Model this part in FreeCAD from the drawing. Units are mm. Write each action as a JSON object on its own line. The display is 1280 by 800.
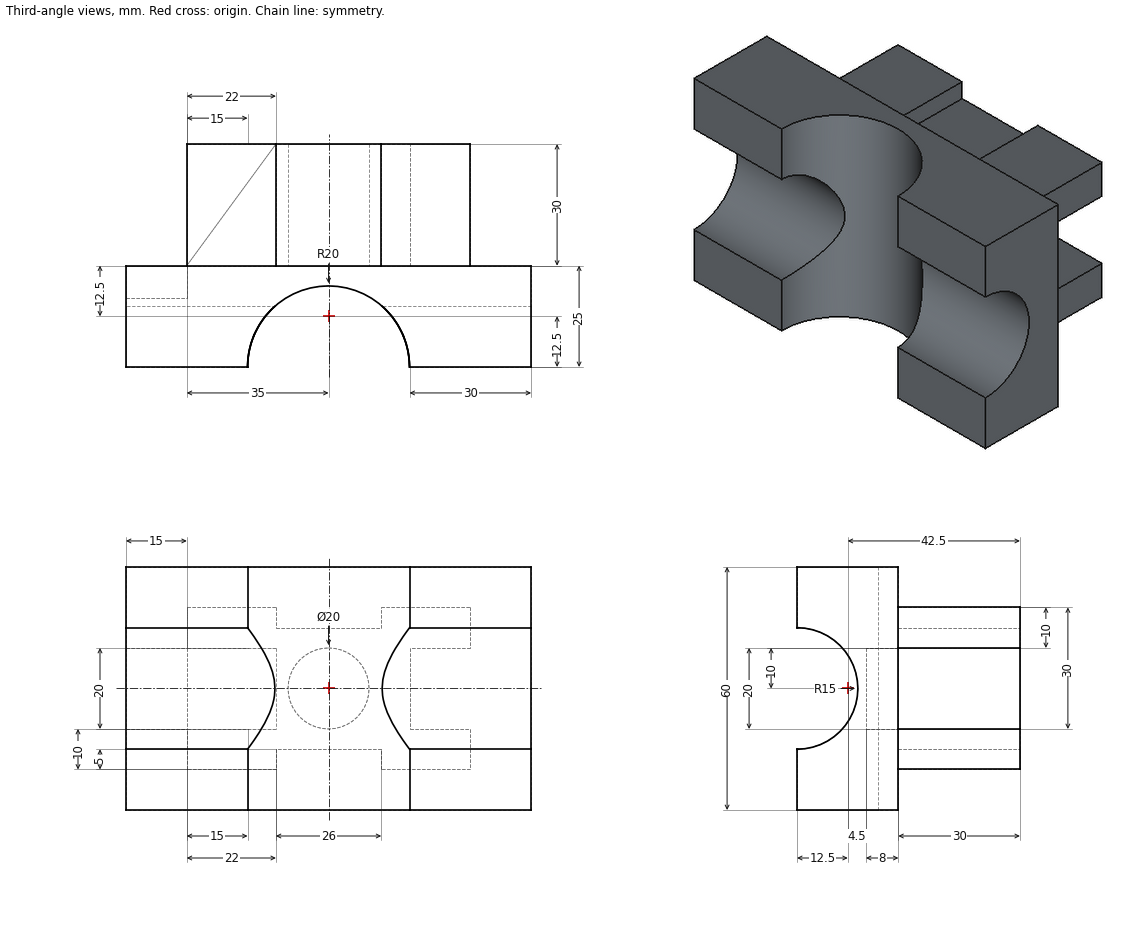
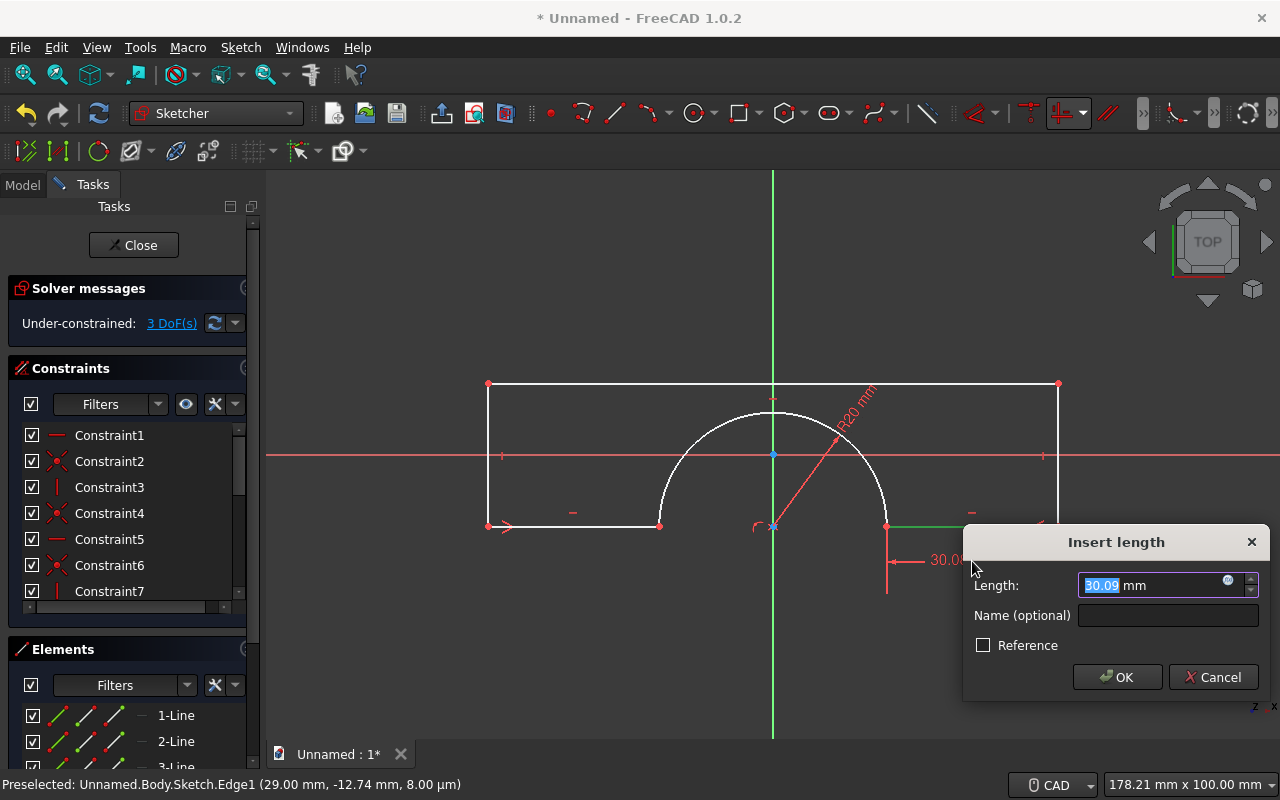
{"action": "type", "text": "30"}
{"action": "key", "text": "Return"}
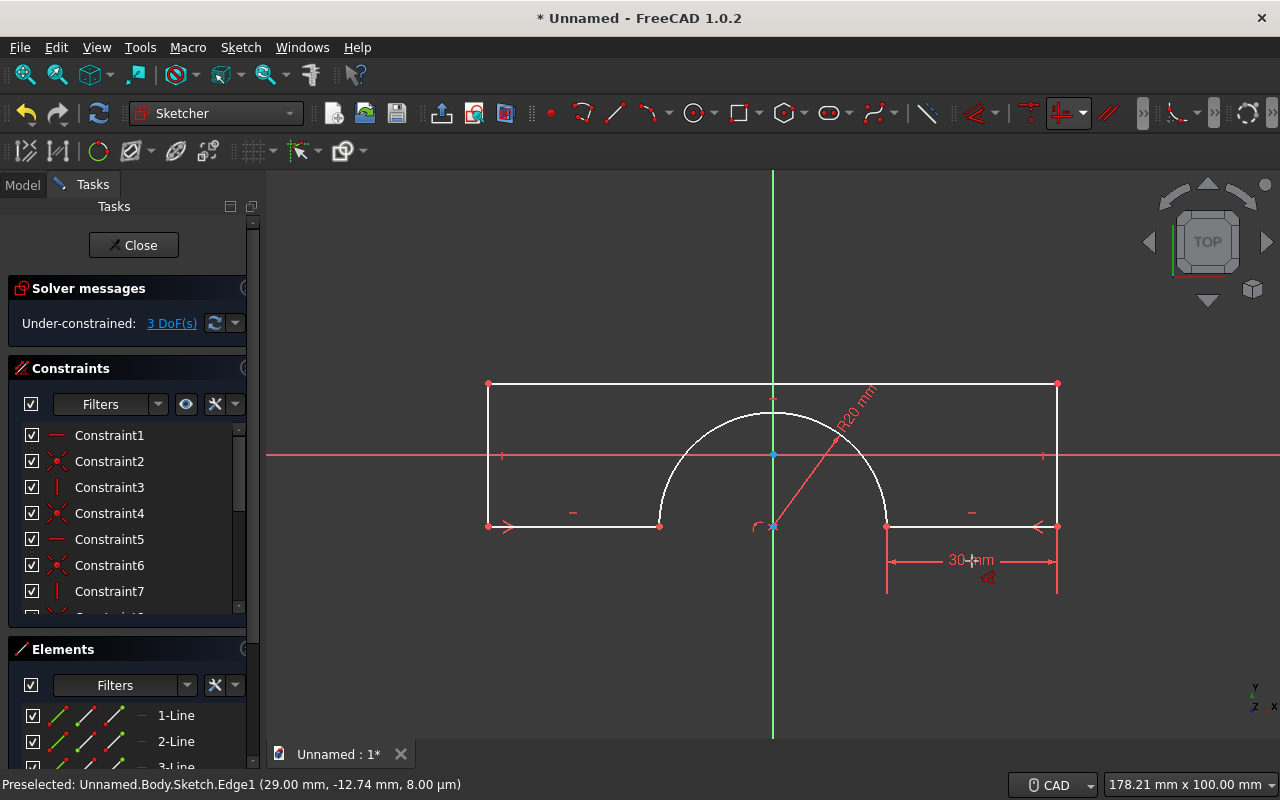
{"action": "left_click", "coordinate": [1057, 484]}
{"action": "left_click", "coordinate": [1091, 423]}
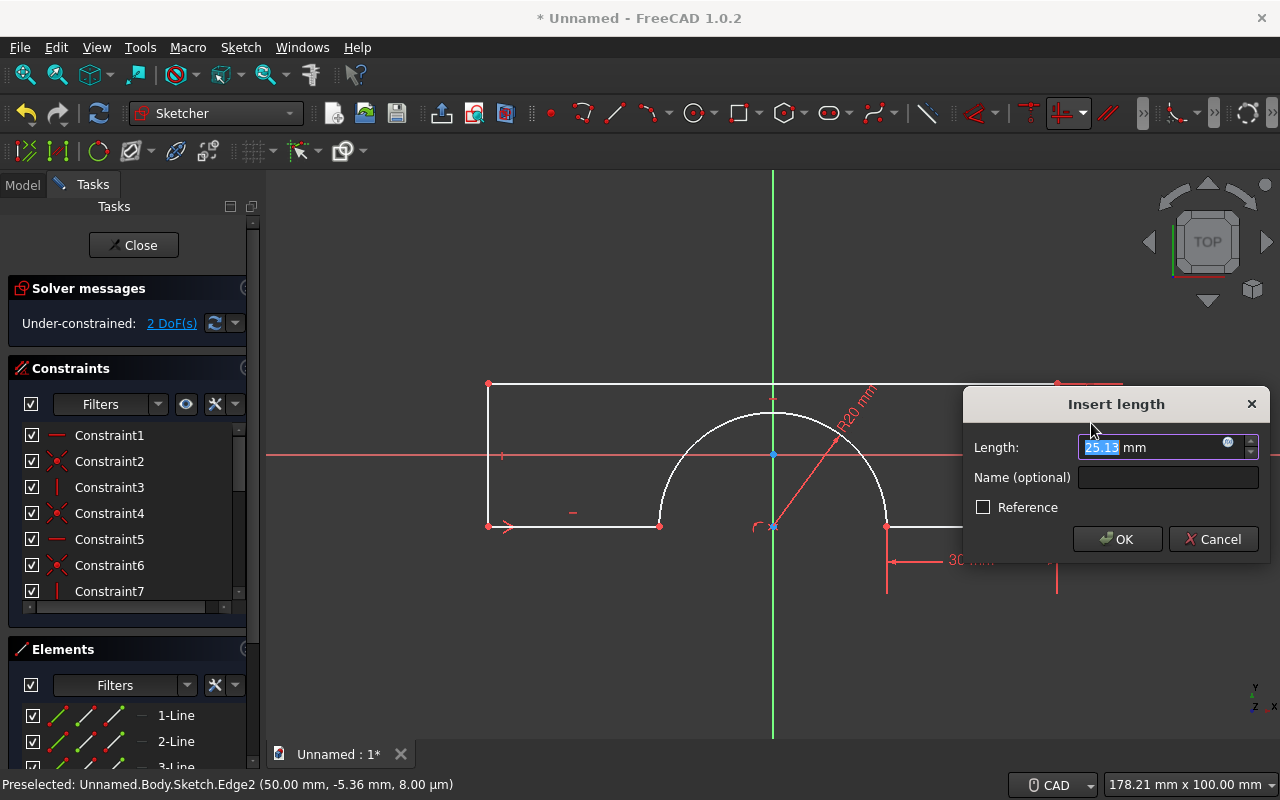
{"action": "type", "text": "25"}
{"action": "key", "text": "Return"}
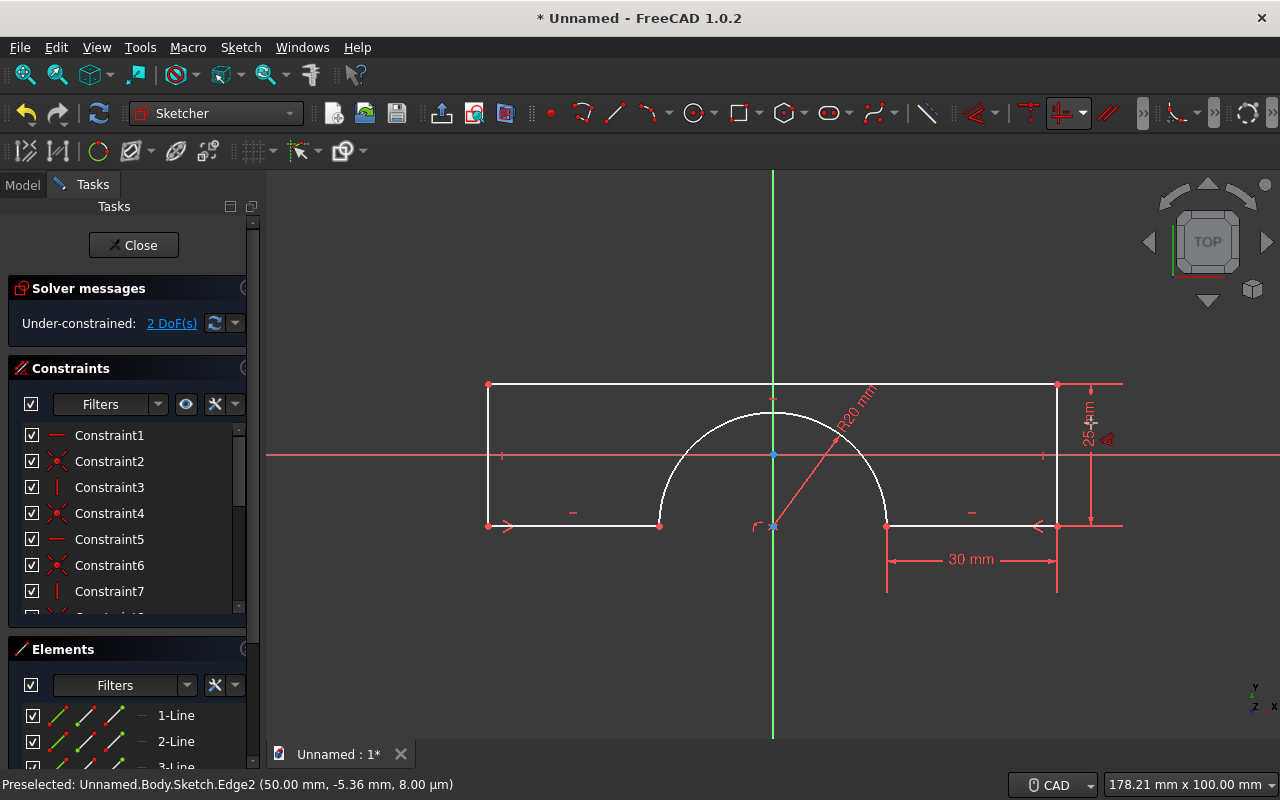
{"action": "left_click", "coordinate": [887, 526]}
{"action": "left_click", "coordinate": [921, 490]}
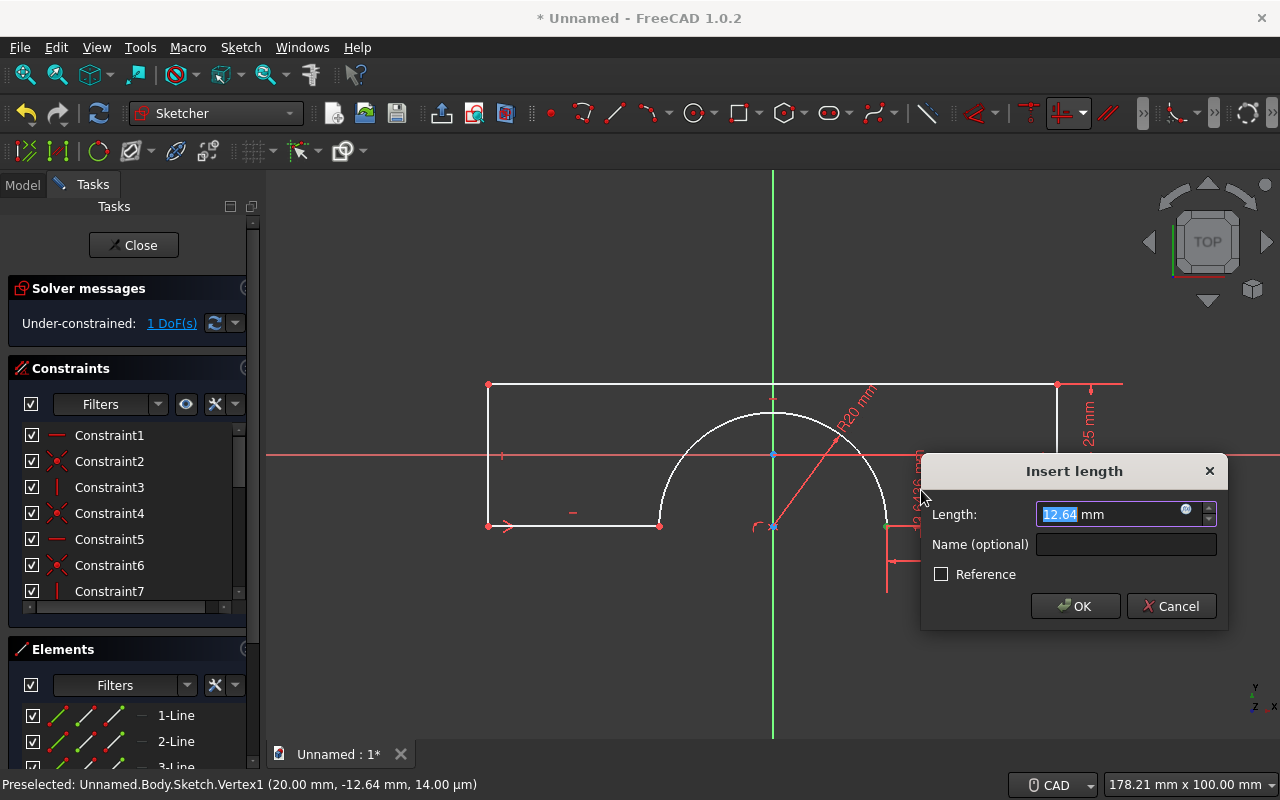
{"action": "type", "text": "12.5"}
{"action": "key", "text": "Return"}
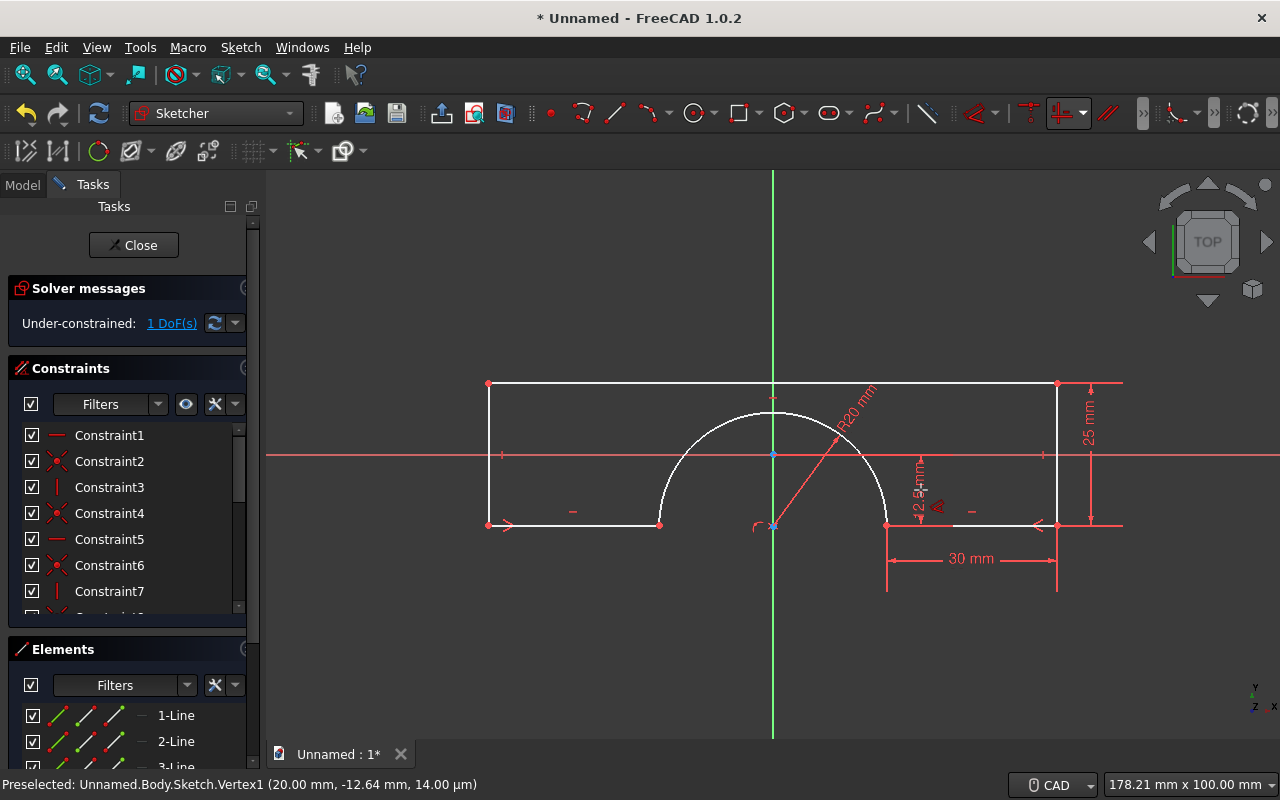
{"action": "left_click", "coordinate": [773, 526]}
{"action": "left_click", "coordinate": [807, 490]}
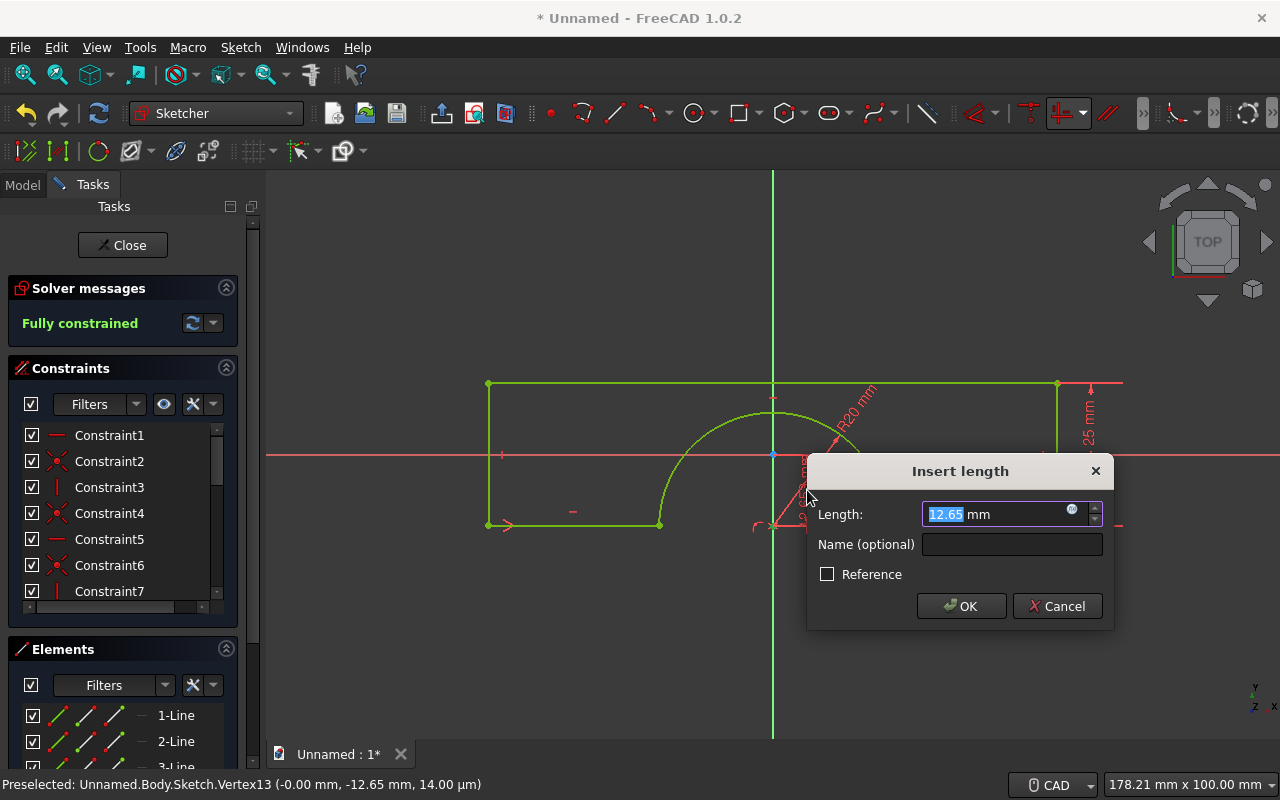
{"action": "type", "text": "12.5"}
{"action": "key", "text": "Return"}
{"action": "key", "text": "Escape"}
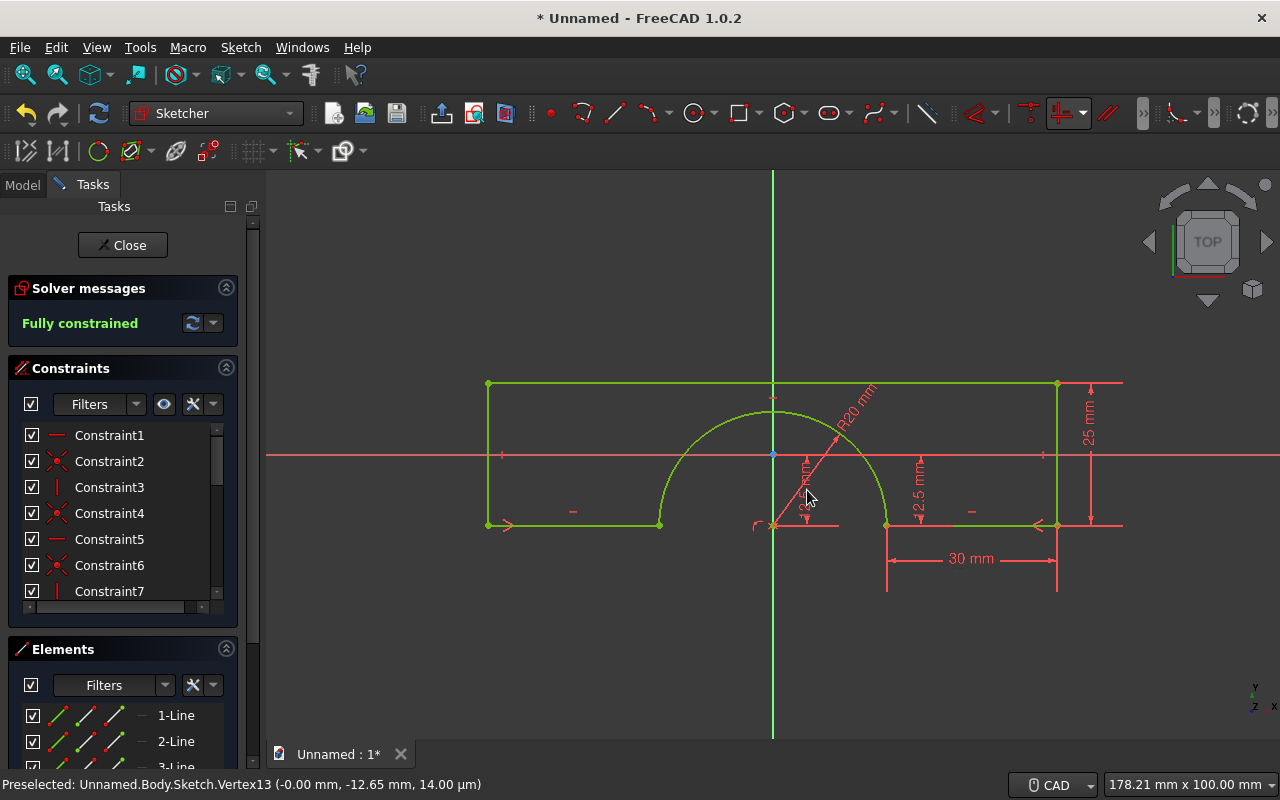
{"action": "left_click", "coordinate": [123, 245]}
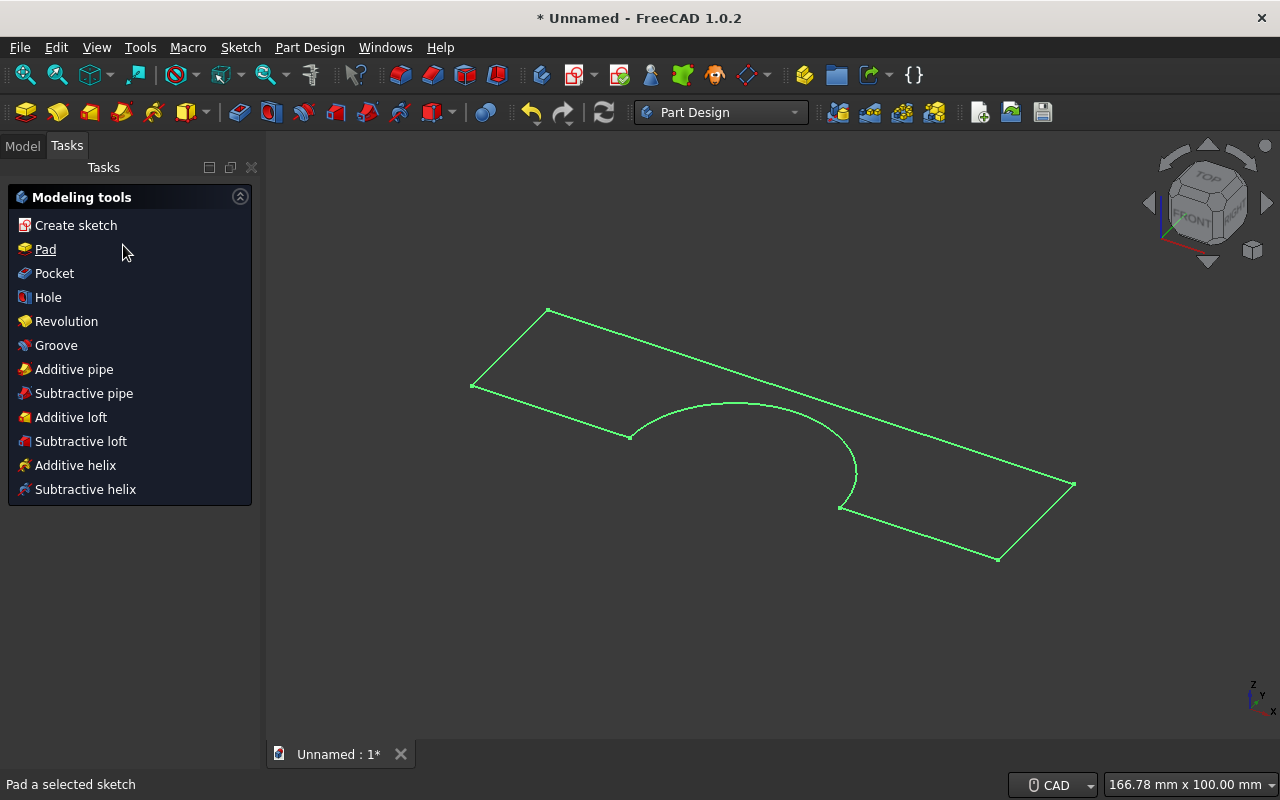
{"action": "left_click", "coordinate": [26, 112]}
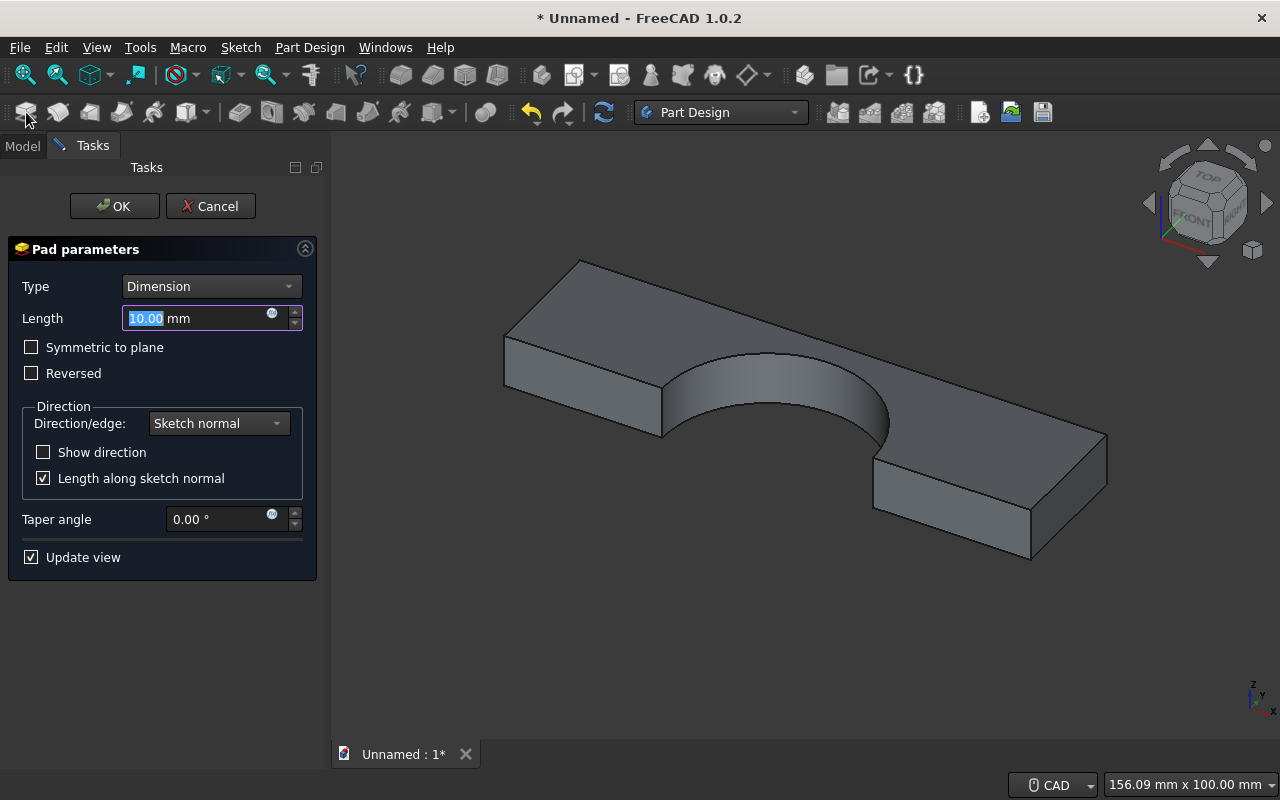
{"action": "type", "text": "60"}
{"action": "key", "text": "Tab"}